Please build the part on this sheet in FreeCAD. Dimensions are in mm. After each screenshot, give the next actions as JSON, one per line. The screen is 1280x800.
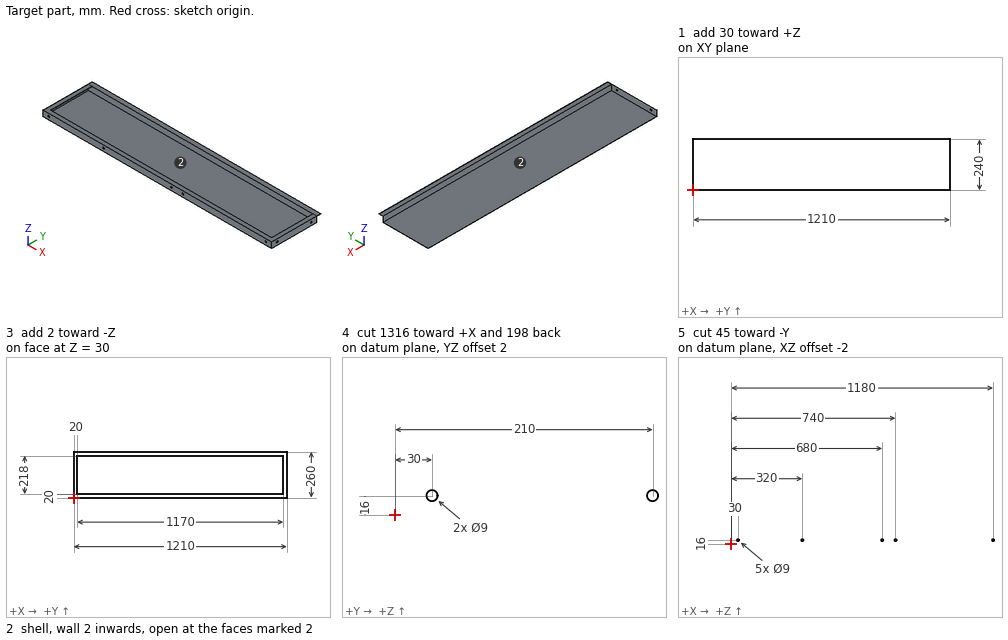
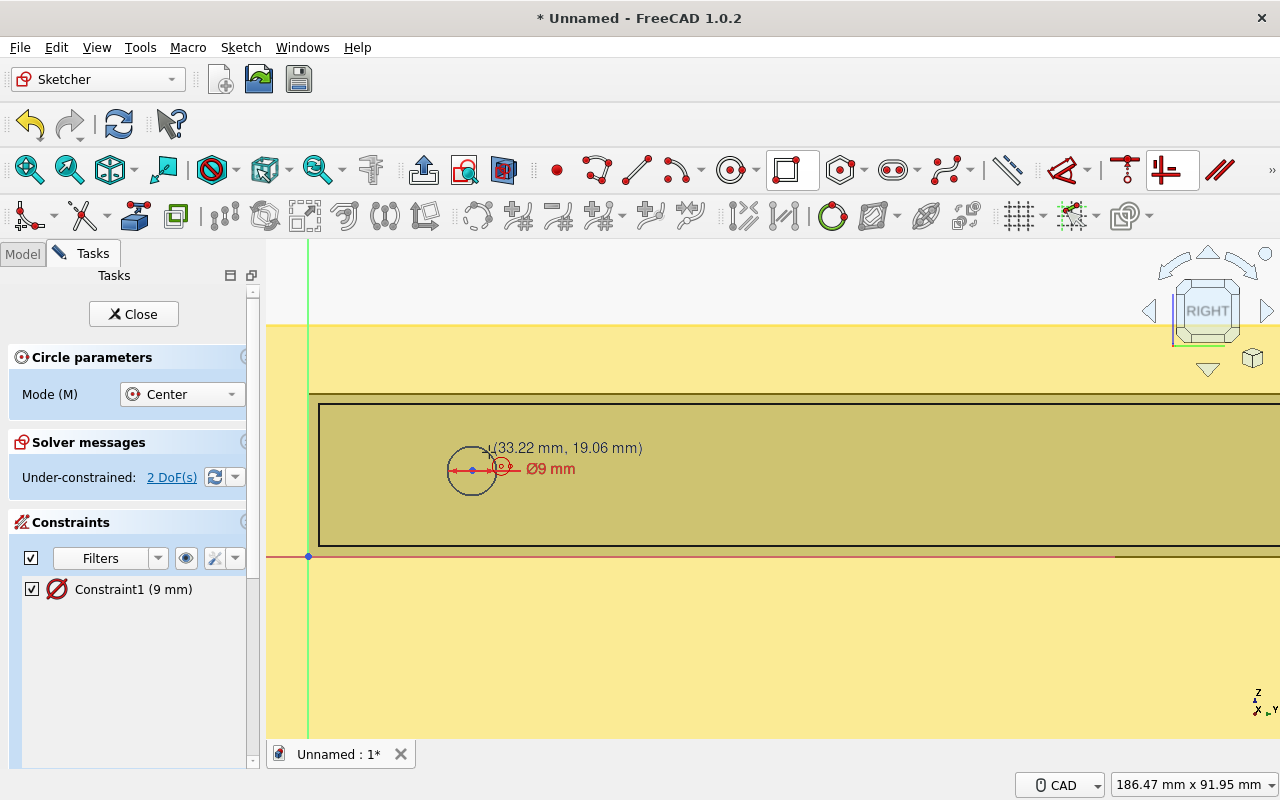
{"action": "scroll", "coordinate": [477, 475], "scroll_direction": "down", "scroll_amount": 3}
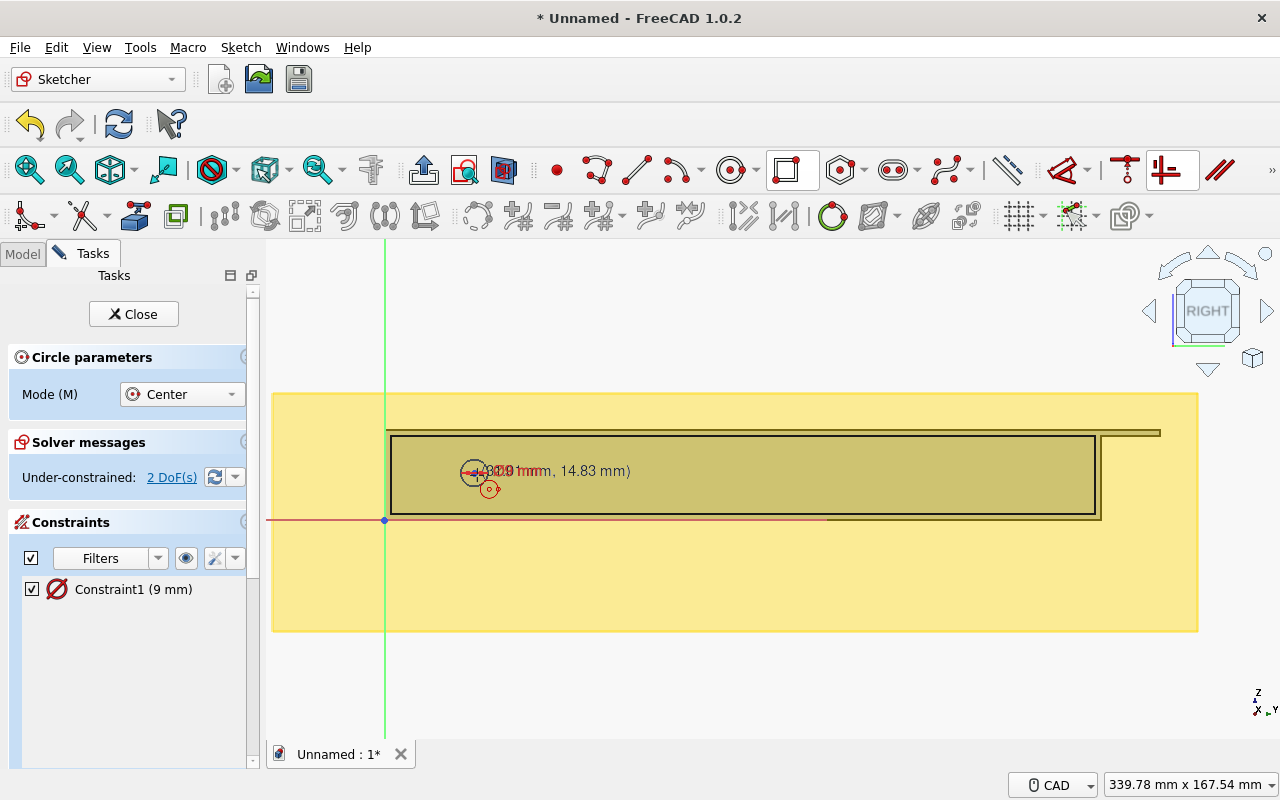
{"action": "scroll", "coordinate": [1011, 472], "scroll_direction": "up", "scroll_amount": 3}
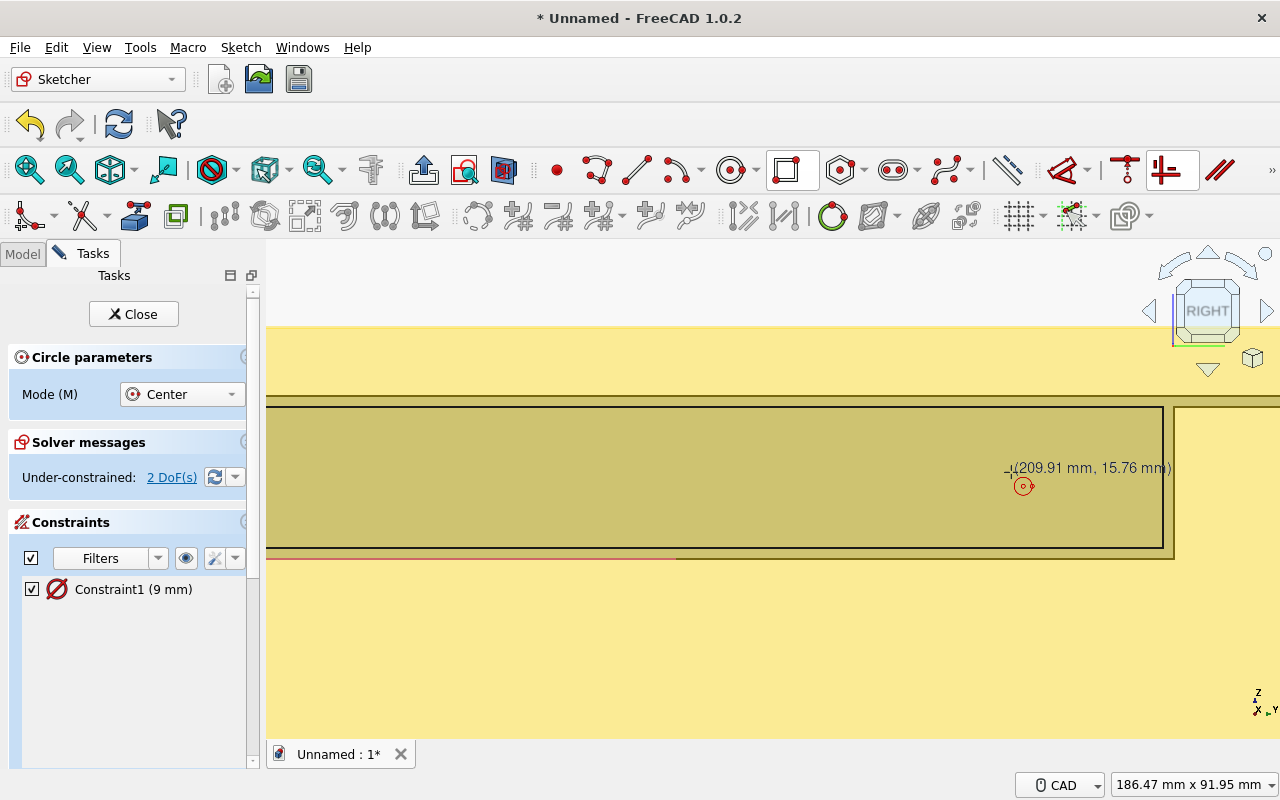
{"action": "left_click", "coordinate": [1011, 472]}
{"action": "mouse_move", "coordinate": [1028, 455]}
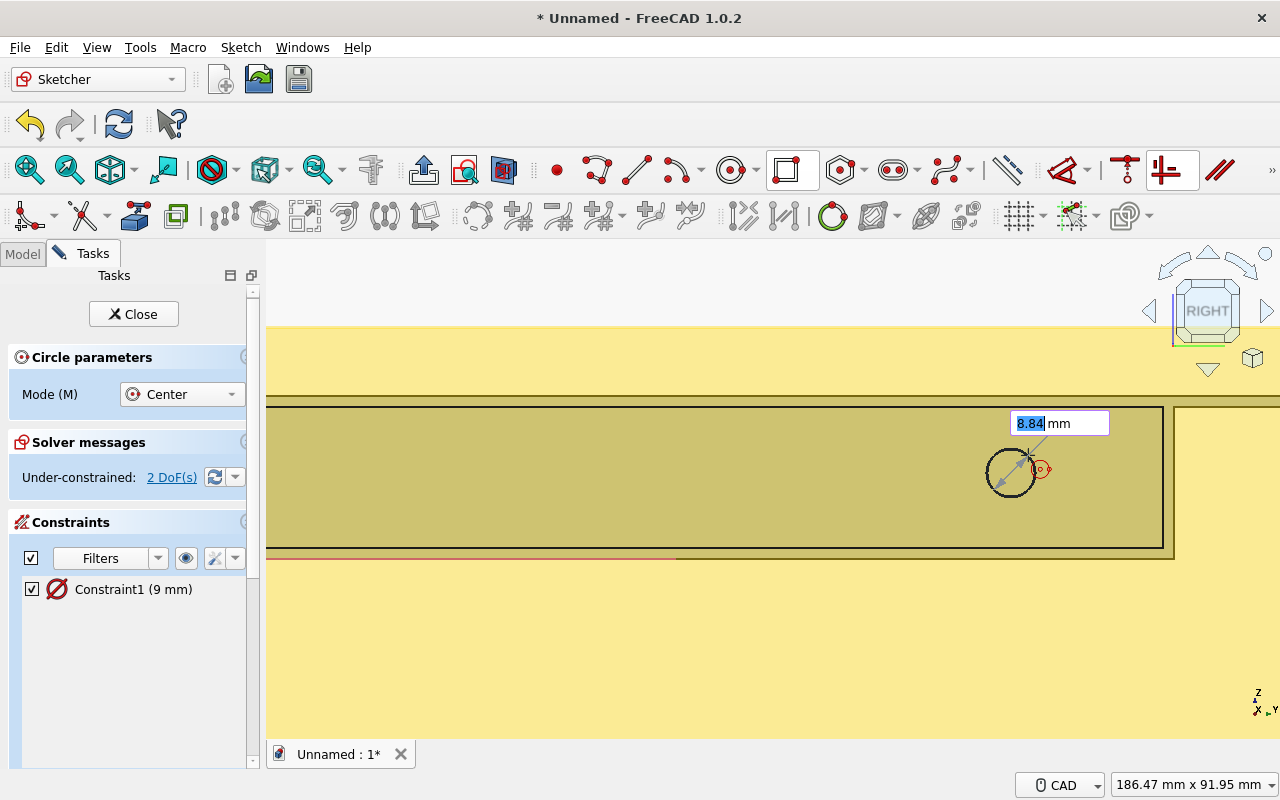
{"action": "type", "text": "9"}
{"action": "key", "text": "Return"}
{"action": "key", "text": "Escape"}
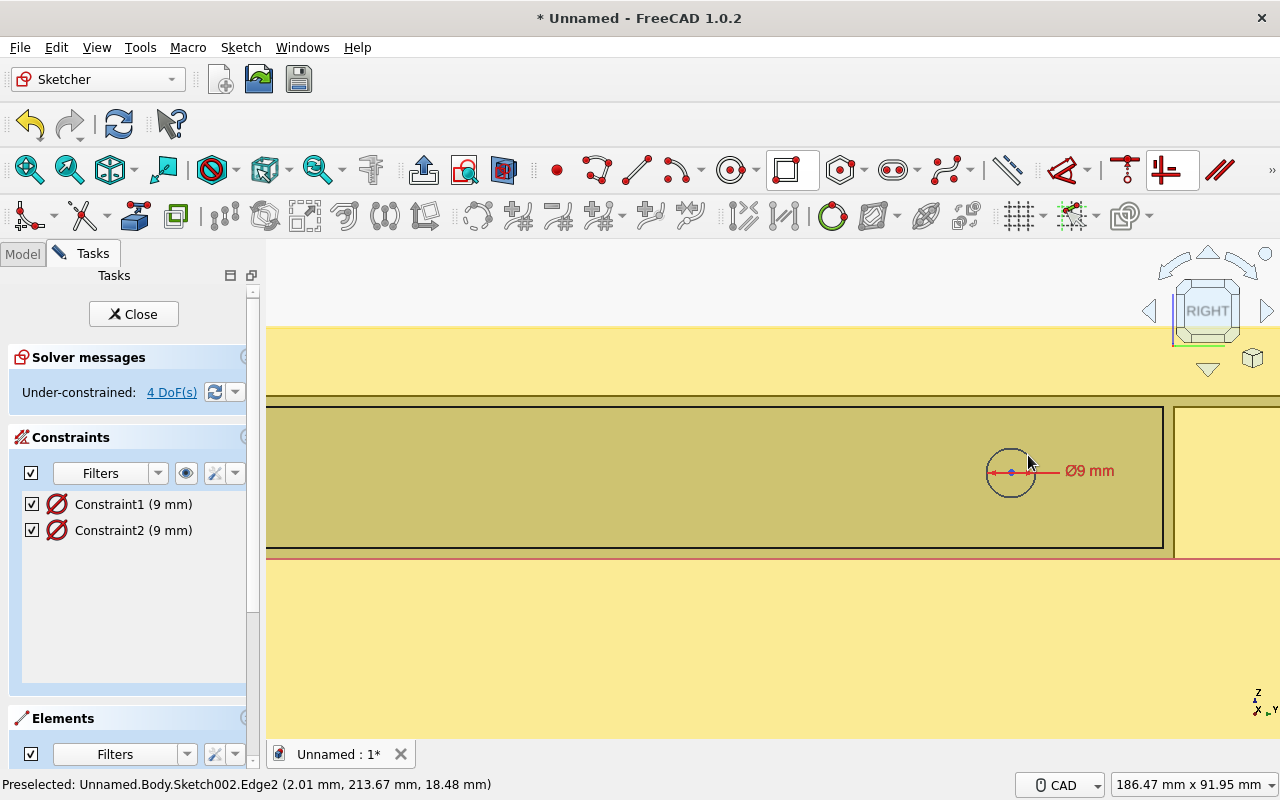
{"action": "scroll", "coordinate": [1011, 472], "scroll_direction": "down", "scroll_amount": 3}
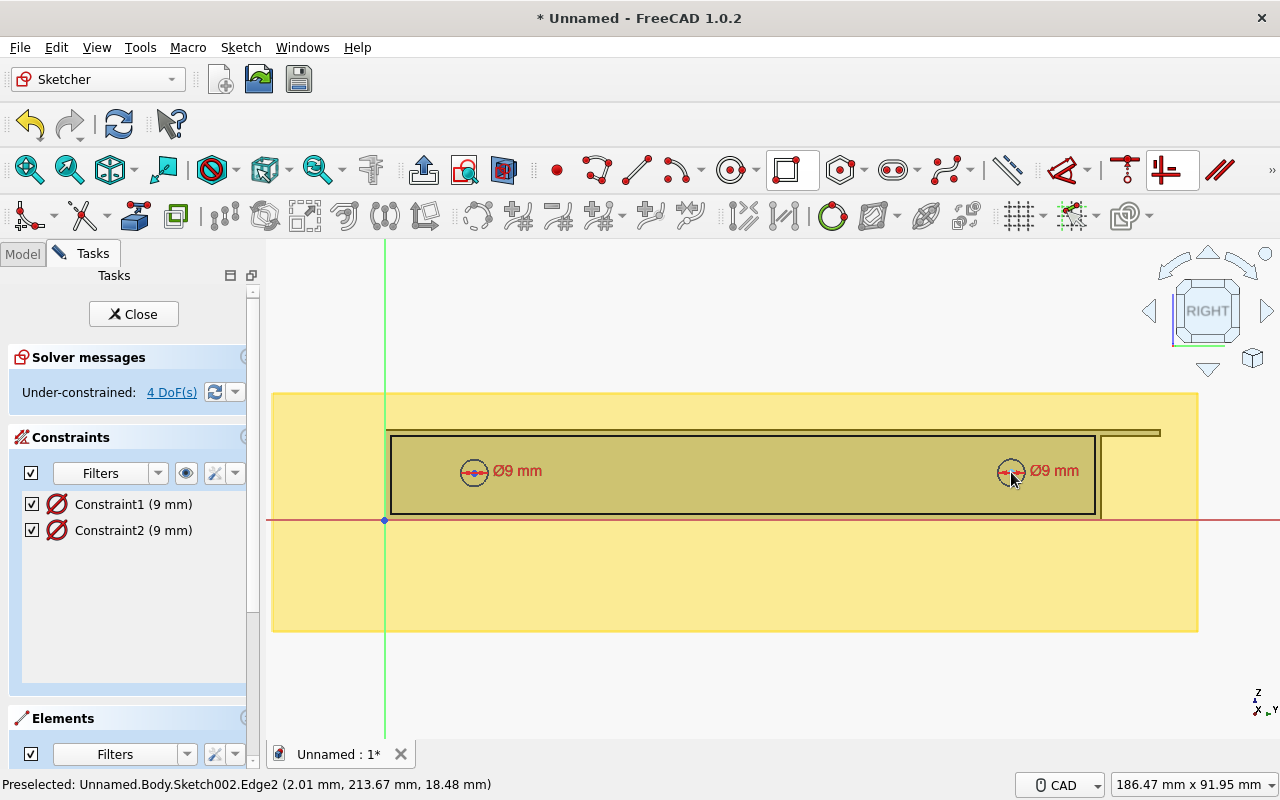
{"action": "left_click", "coordinate": [474, 473]}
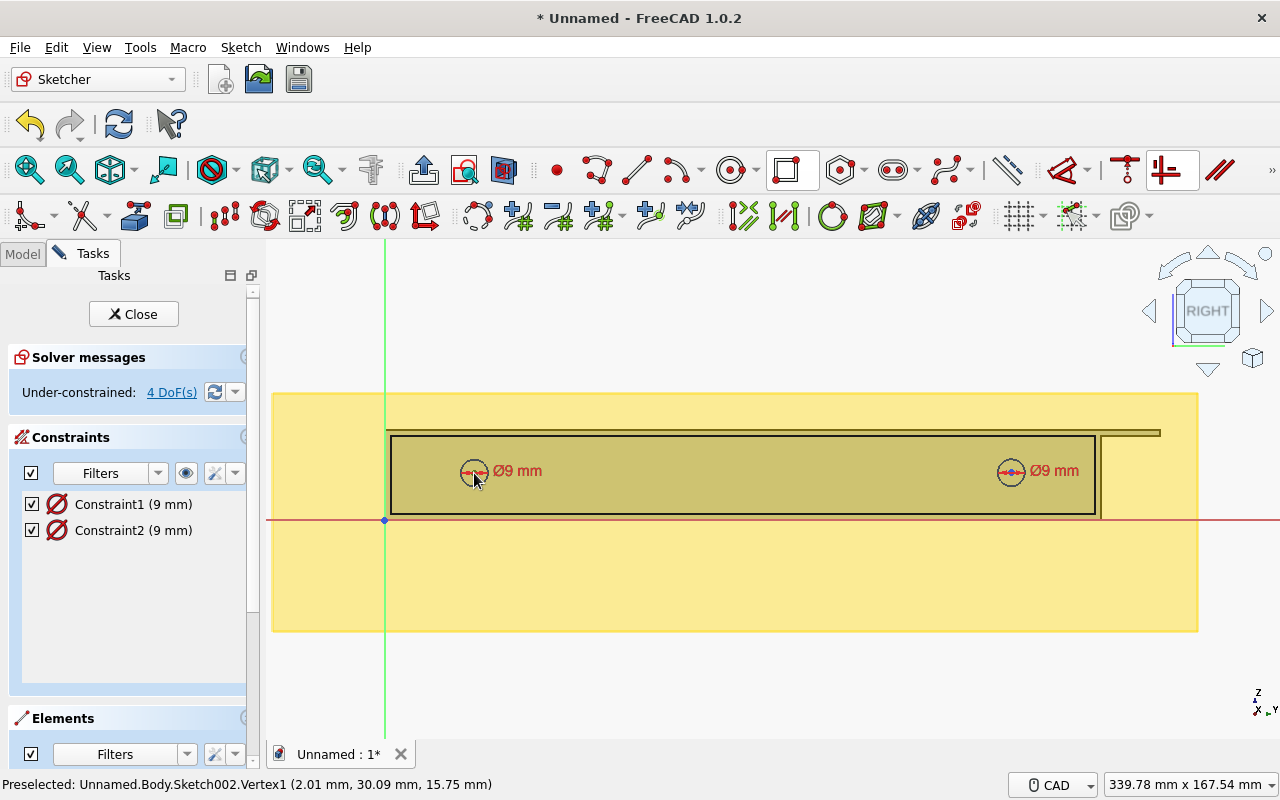
{"action": "left_click", "coordinate": [1011, 473]}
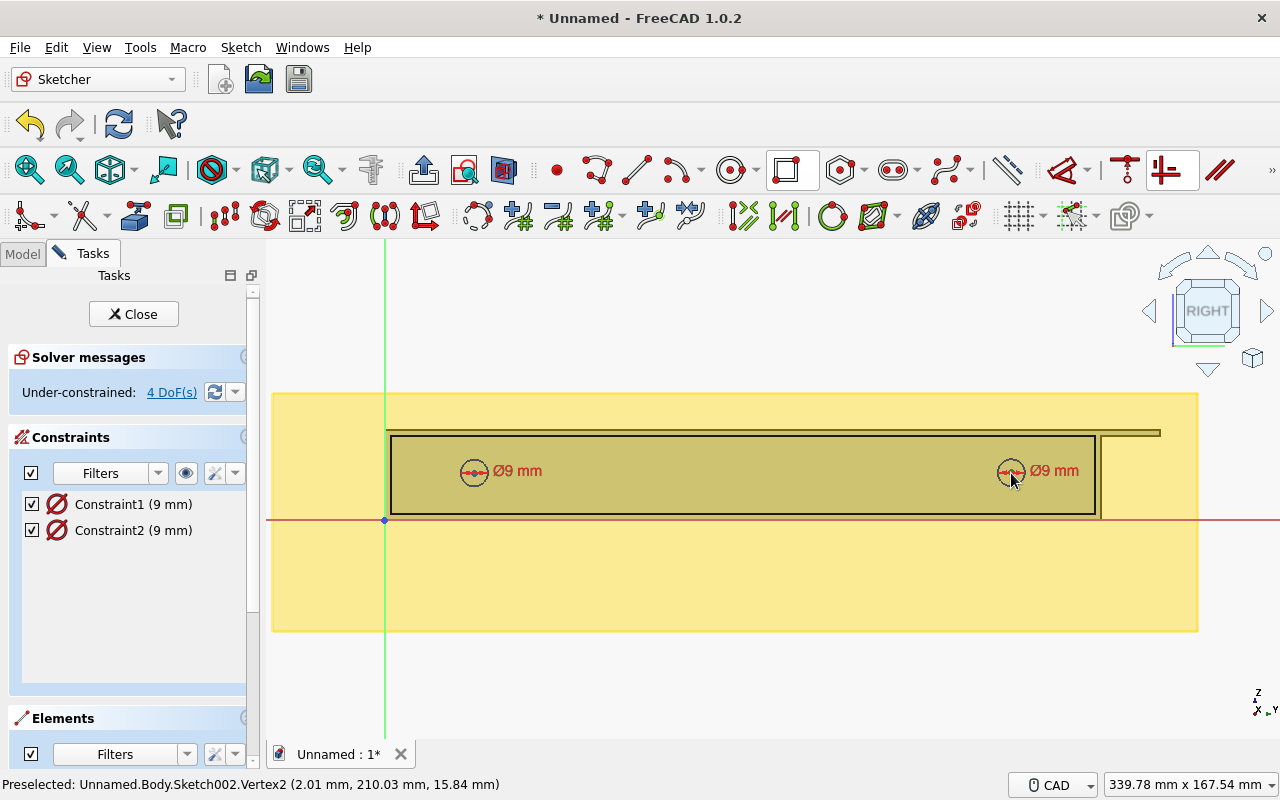
{"action": "left_click", "coordinate": [1194, 170]}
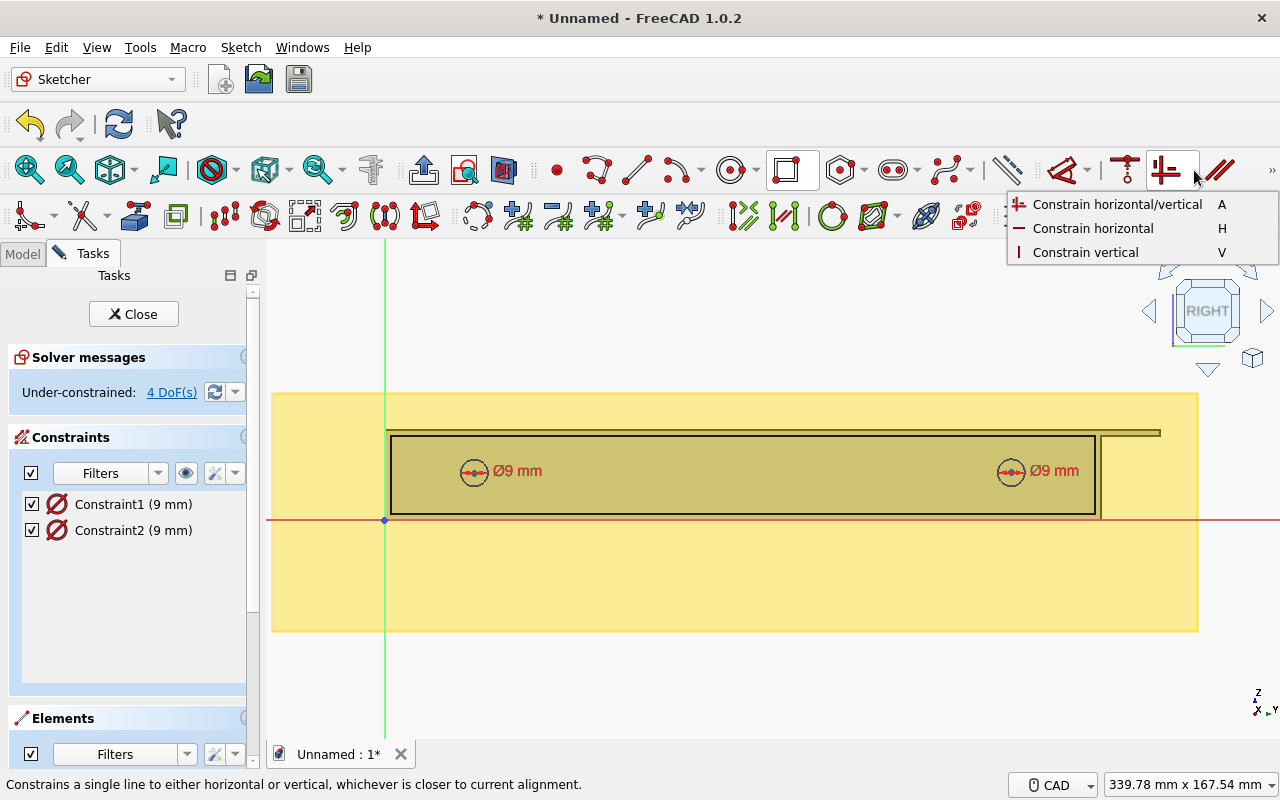
{"action": "left_click", "coordinate": [1143, 228]}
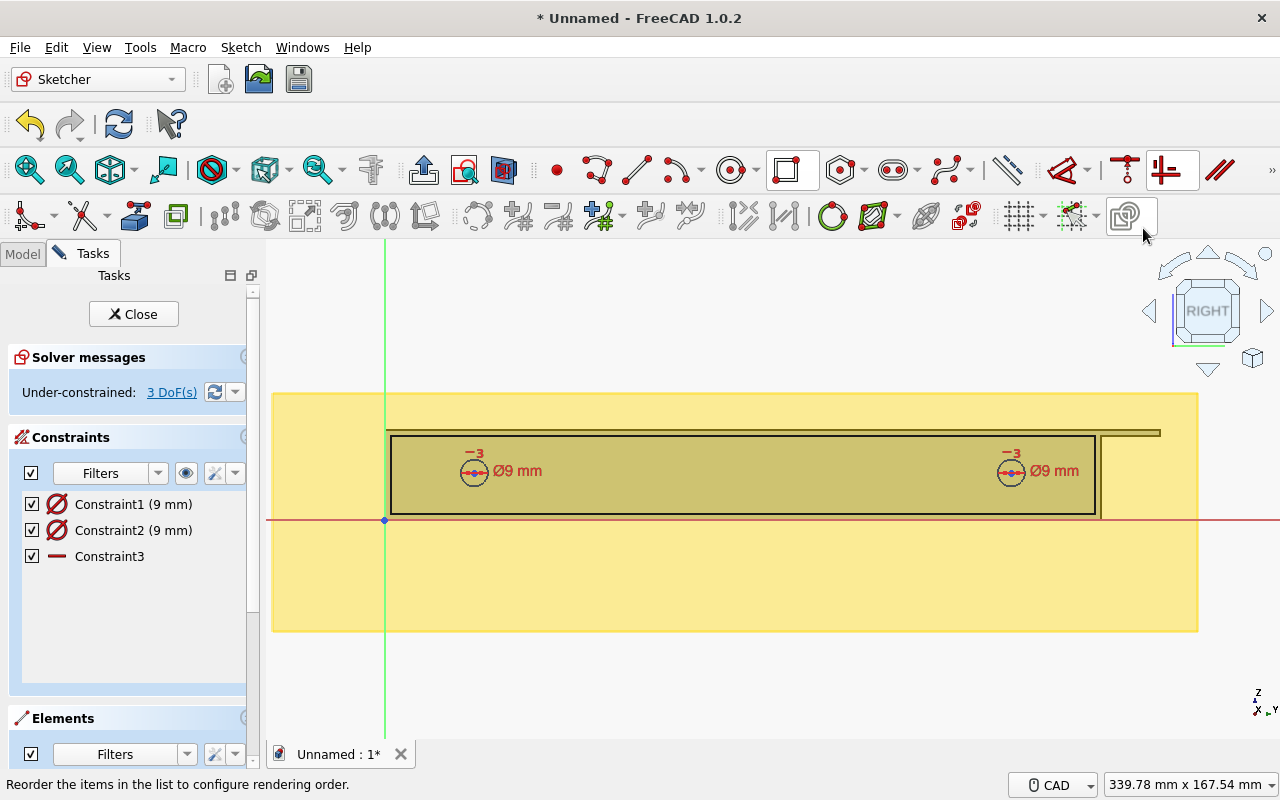
{"action": "left_click", "coordinate": [1062, 170]}